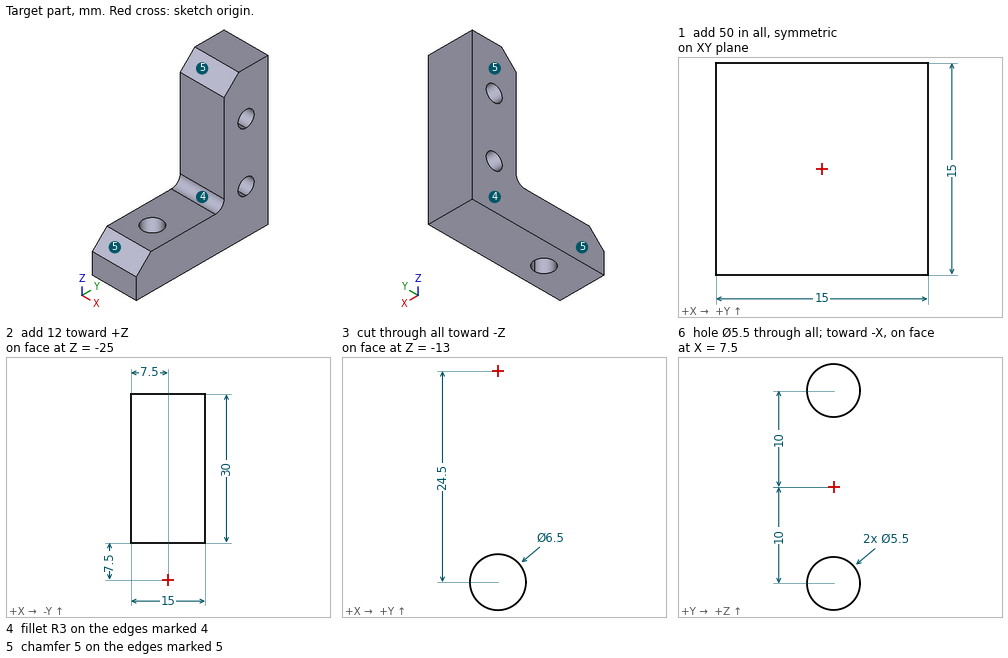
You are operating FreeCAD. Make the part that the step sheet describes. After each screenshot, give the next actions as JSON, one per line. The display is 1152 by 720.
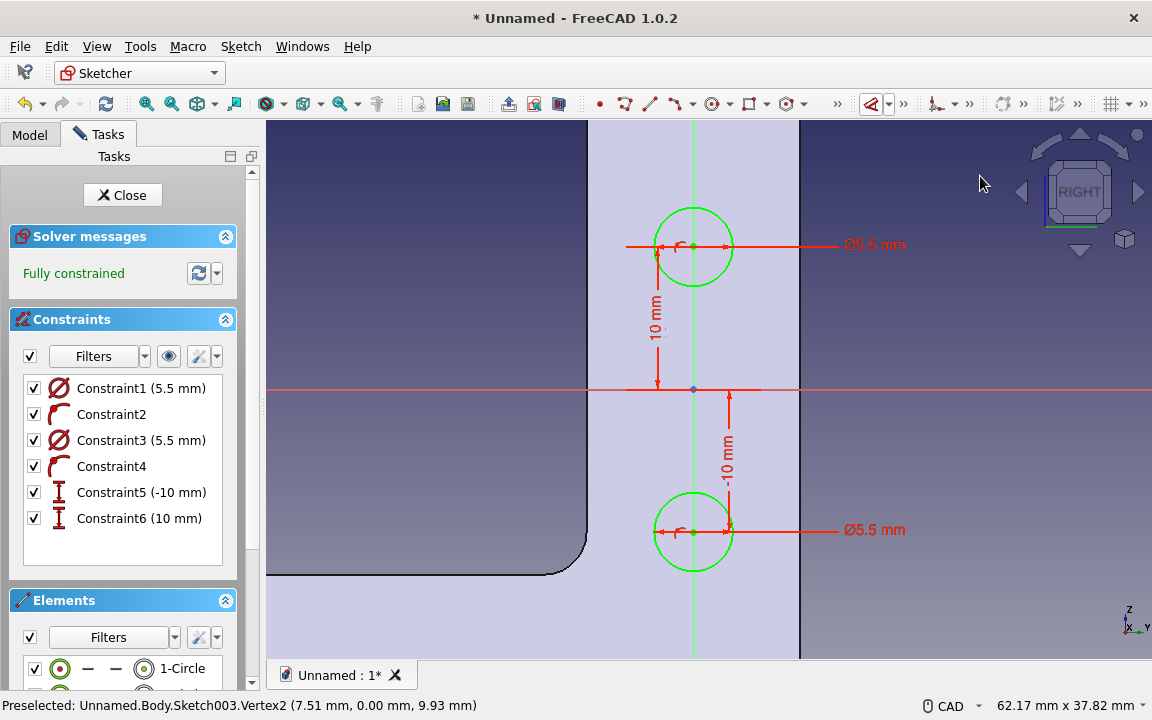
{"action": "left_click", "coordinate": [123, 195]}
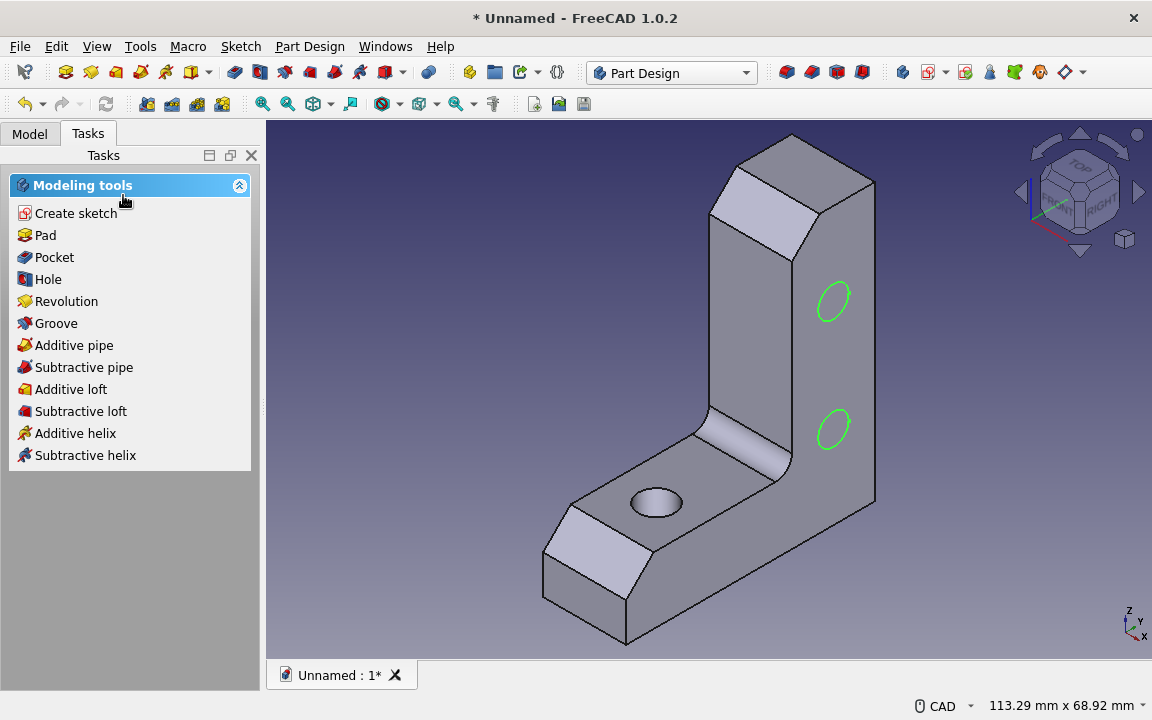
{"action": "left_click", "coordinate": [260, 72]}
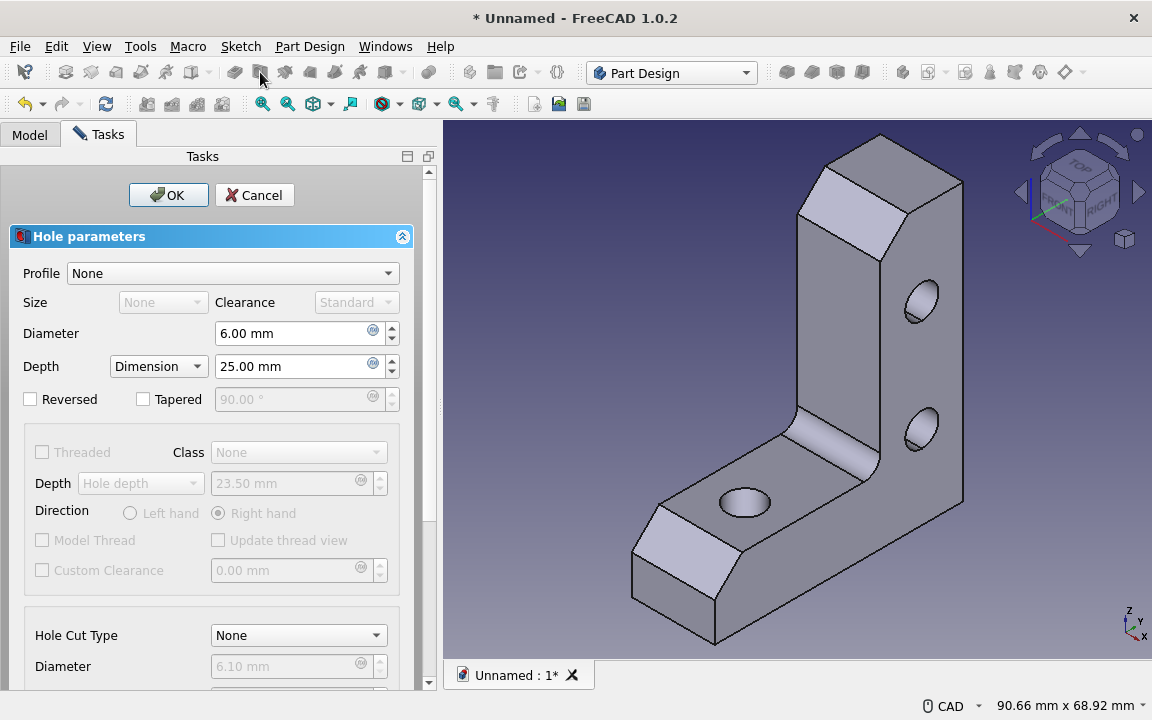
{"action": "triple_click", "coordinate": [300, 334]}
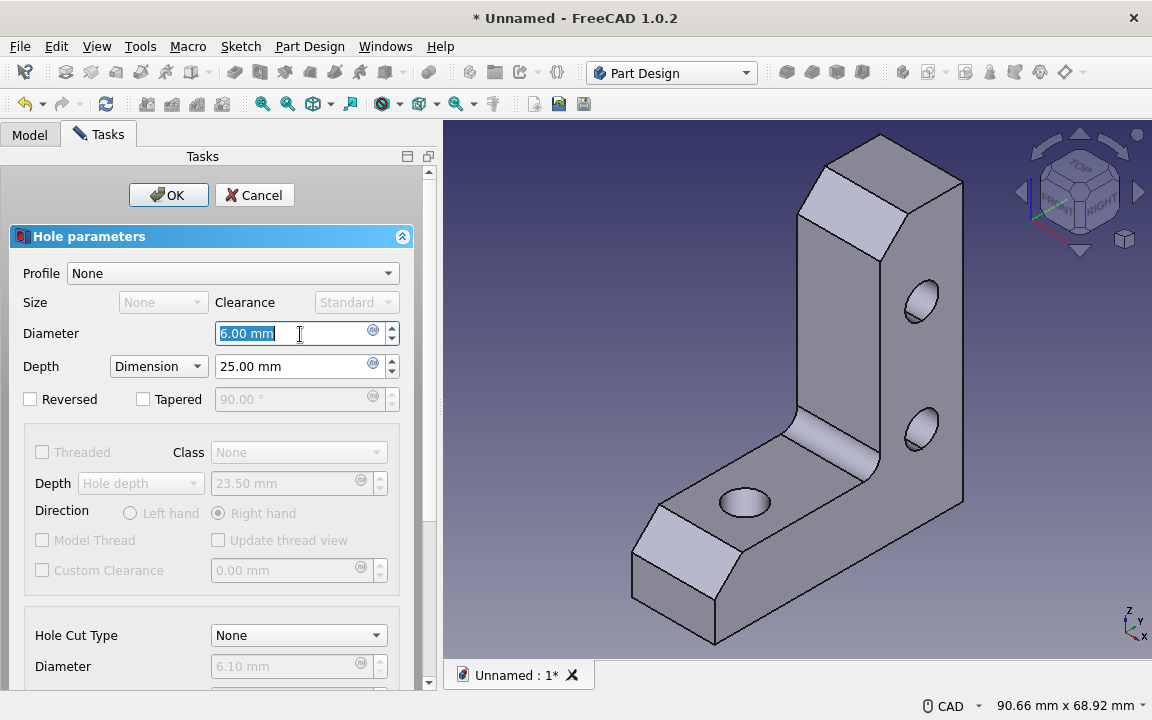
{"action": "type", "text": "5.5"}
{"action": "key", "text": "Tab"}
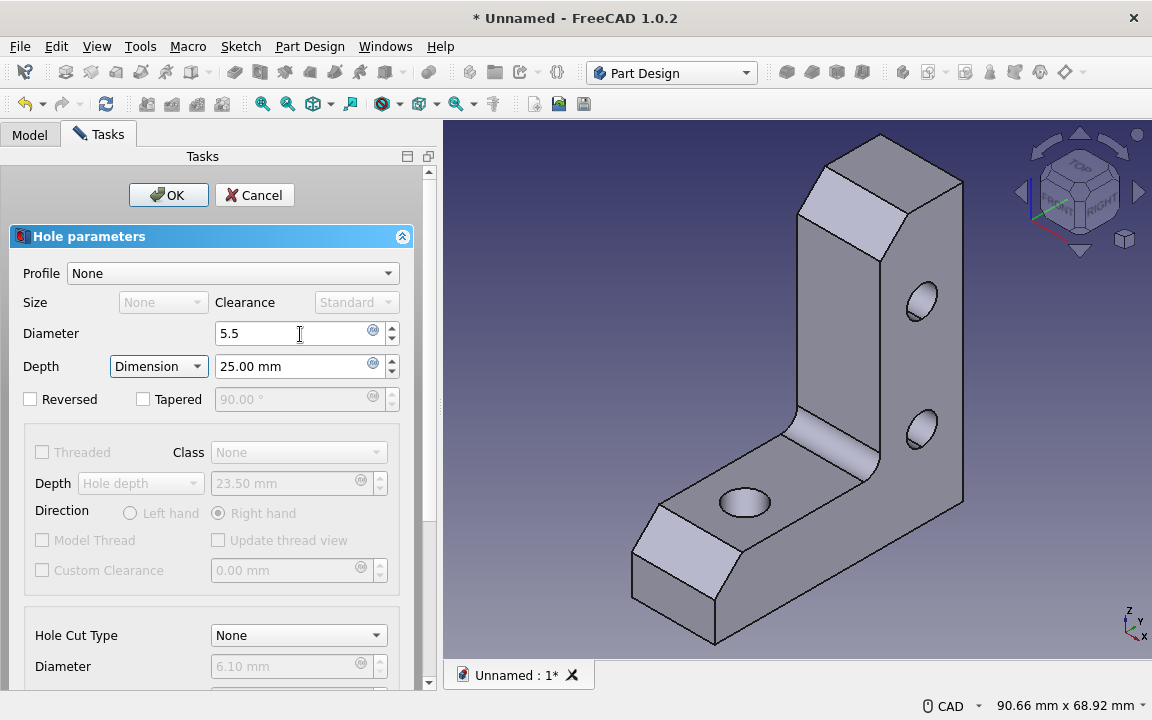
{"action": "left_click", "coordinate": [160, 366]}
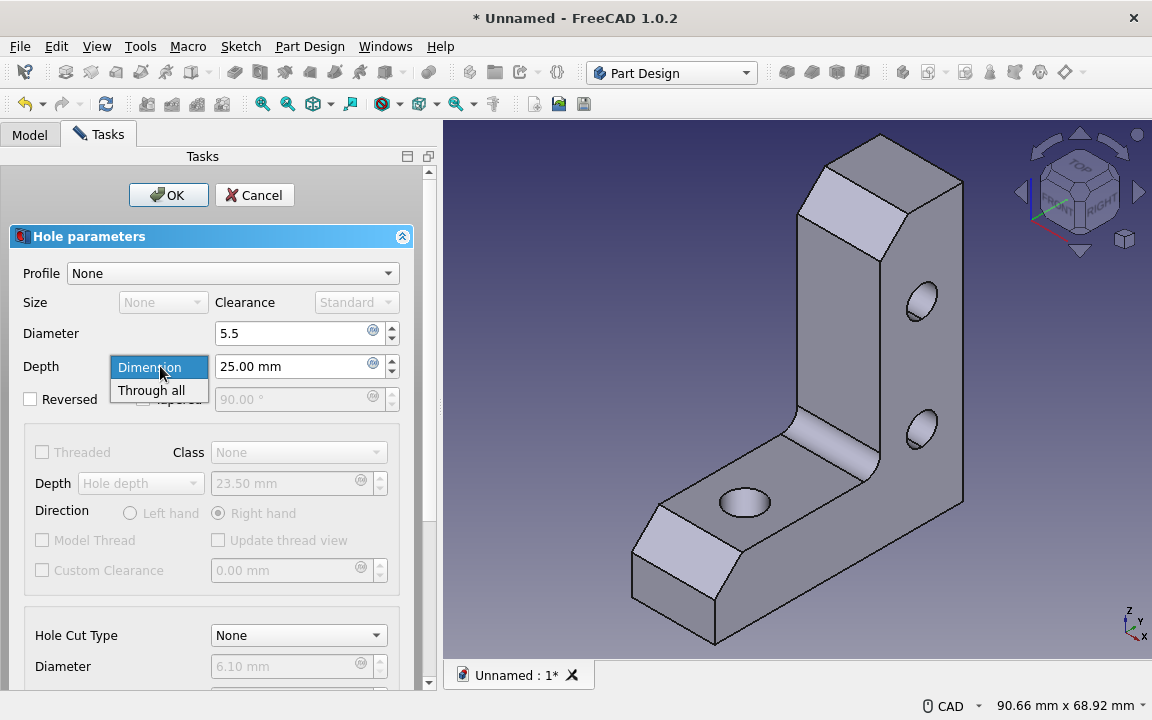
{"action": "left_click", "coordinate": [158, 390]}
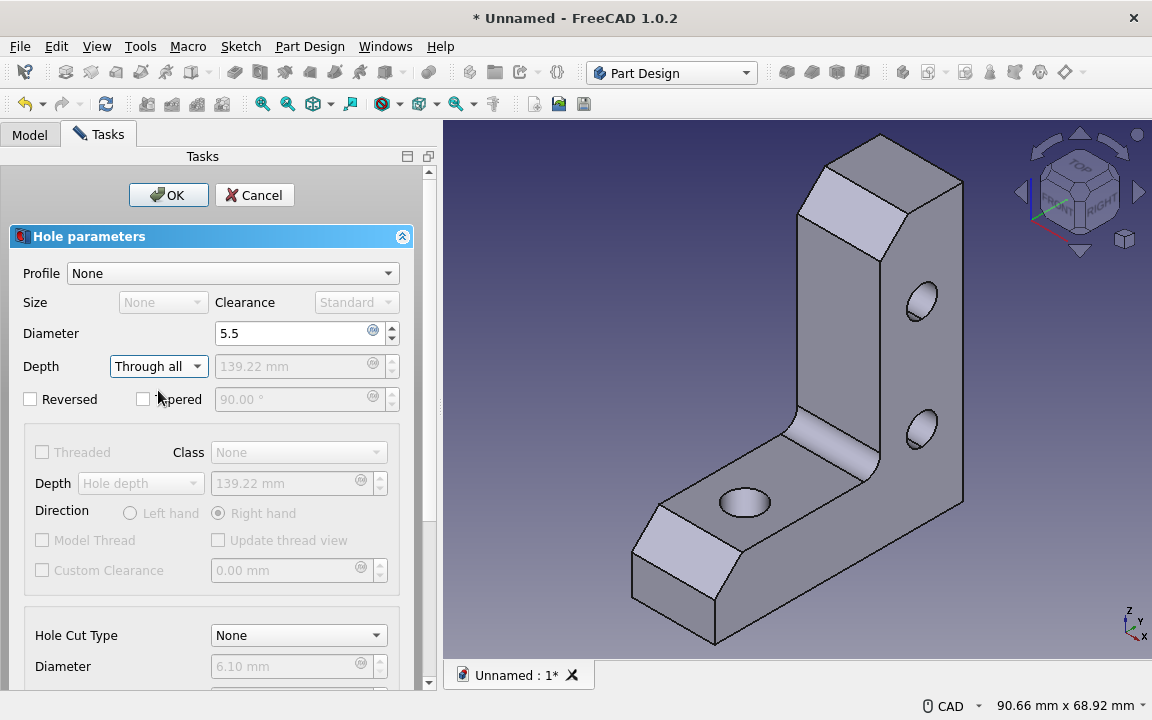
{"action": "left_click", "coordinate": [169, 195]}